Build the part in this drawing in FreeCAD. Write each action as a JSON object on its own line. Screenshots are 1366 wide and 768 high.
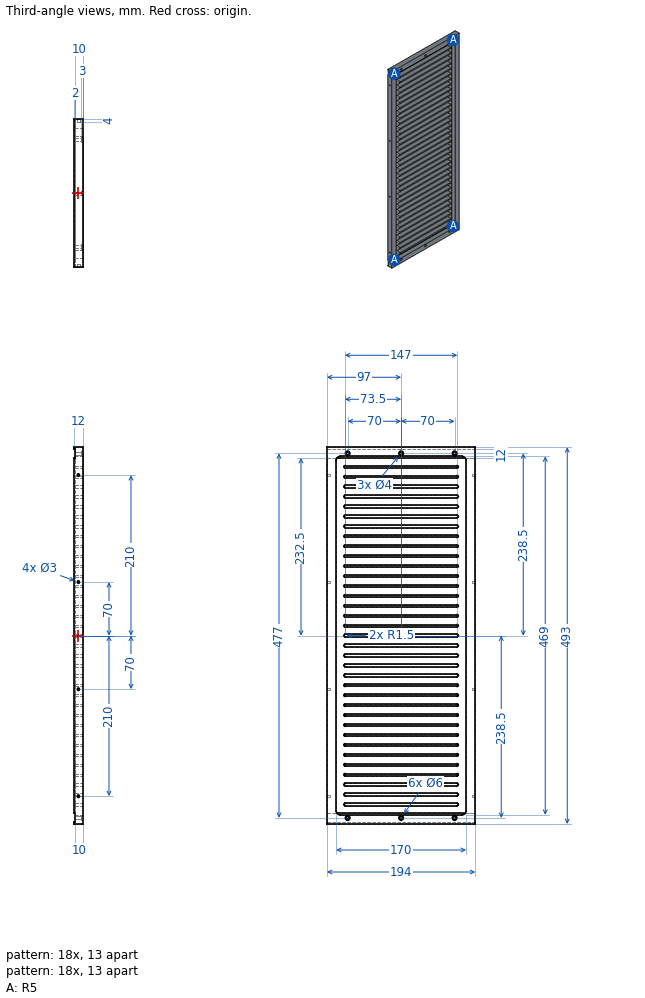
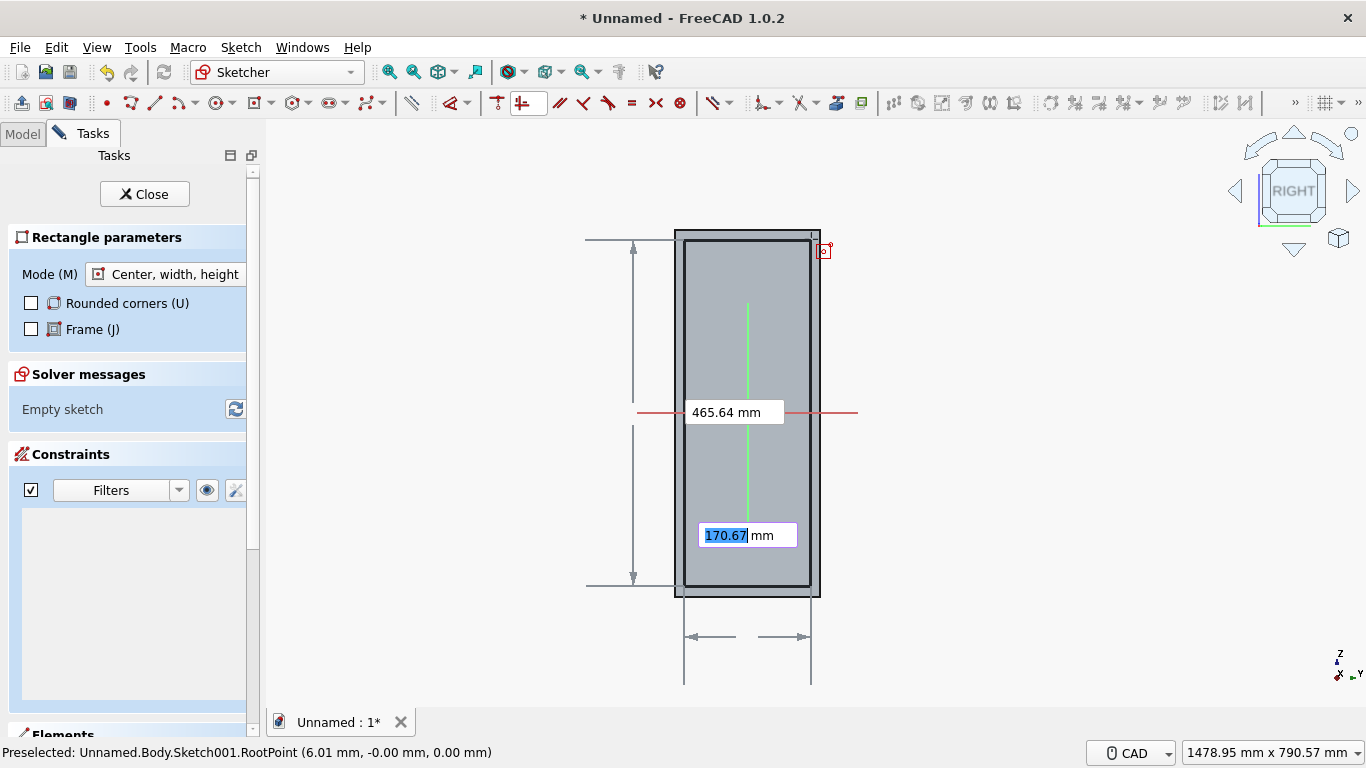
{"action": "type", "text": "170"}
{"action": "key", "text": "Tab"}
{"action": "type", "text": "469"}
{"action": "key", "text": "Return"}
{"action": "key", "text": "Escape"}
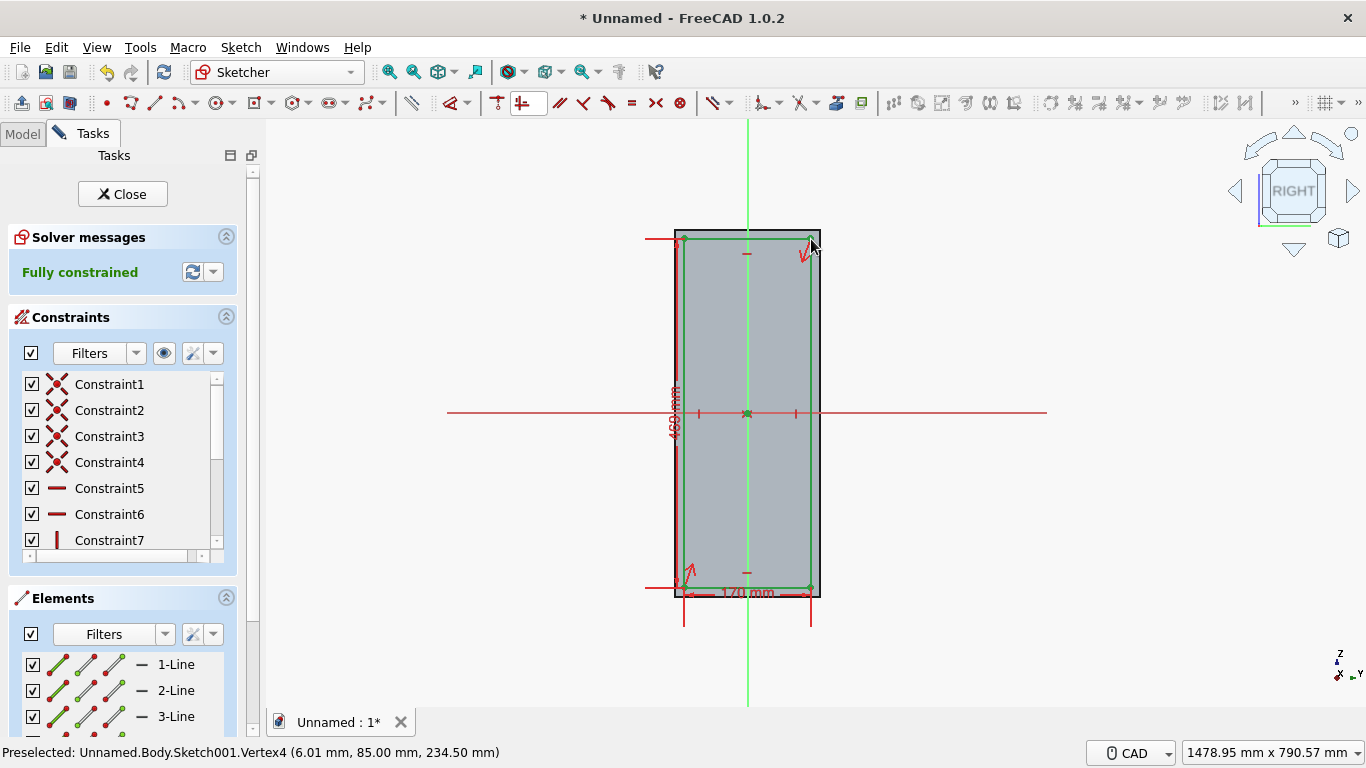
{"action": "left_click", "coordinate": [123, 194]}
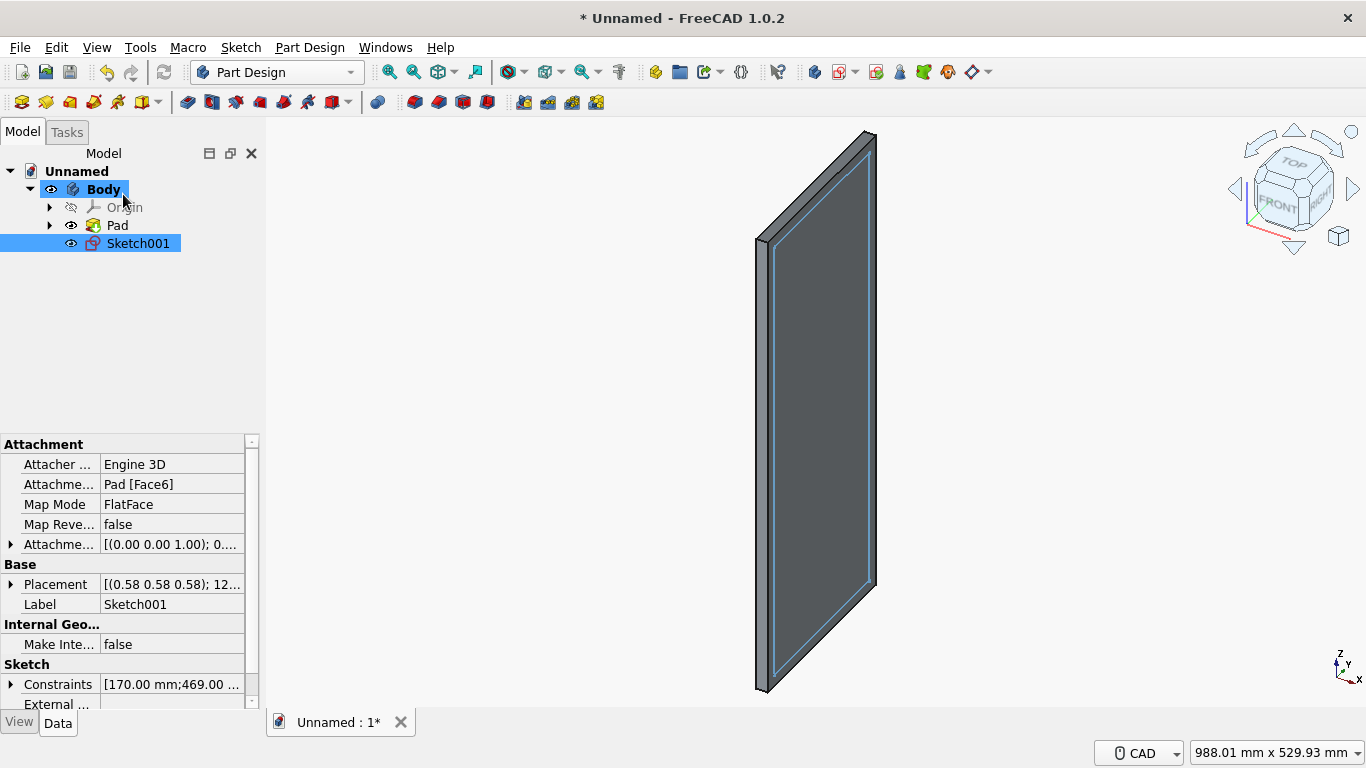
{"action": "left_click", "coordinate": [188, 102]}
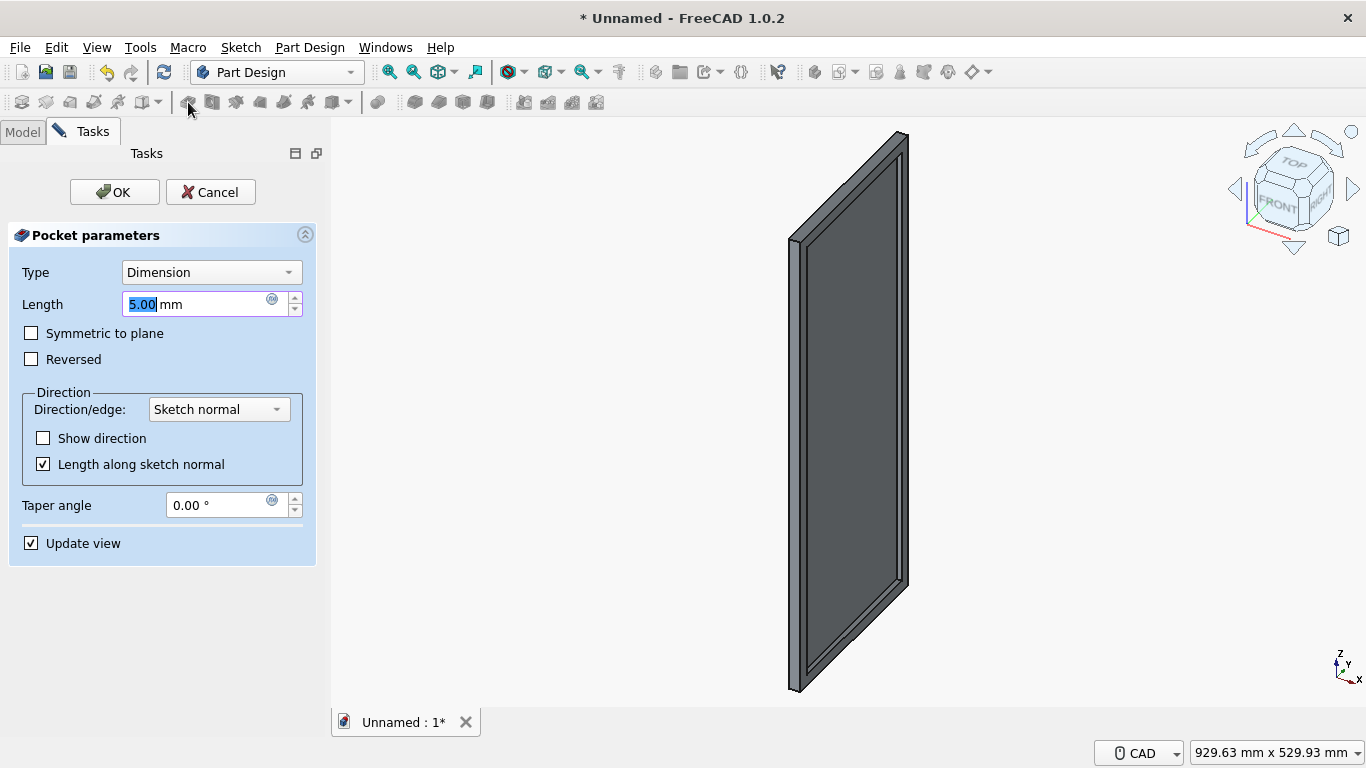
{"action": "type", "text": "10"}
{"action": "key", "text": "Tab"}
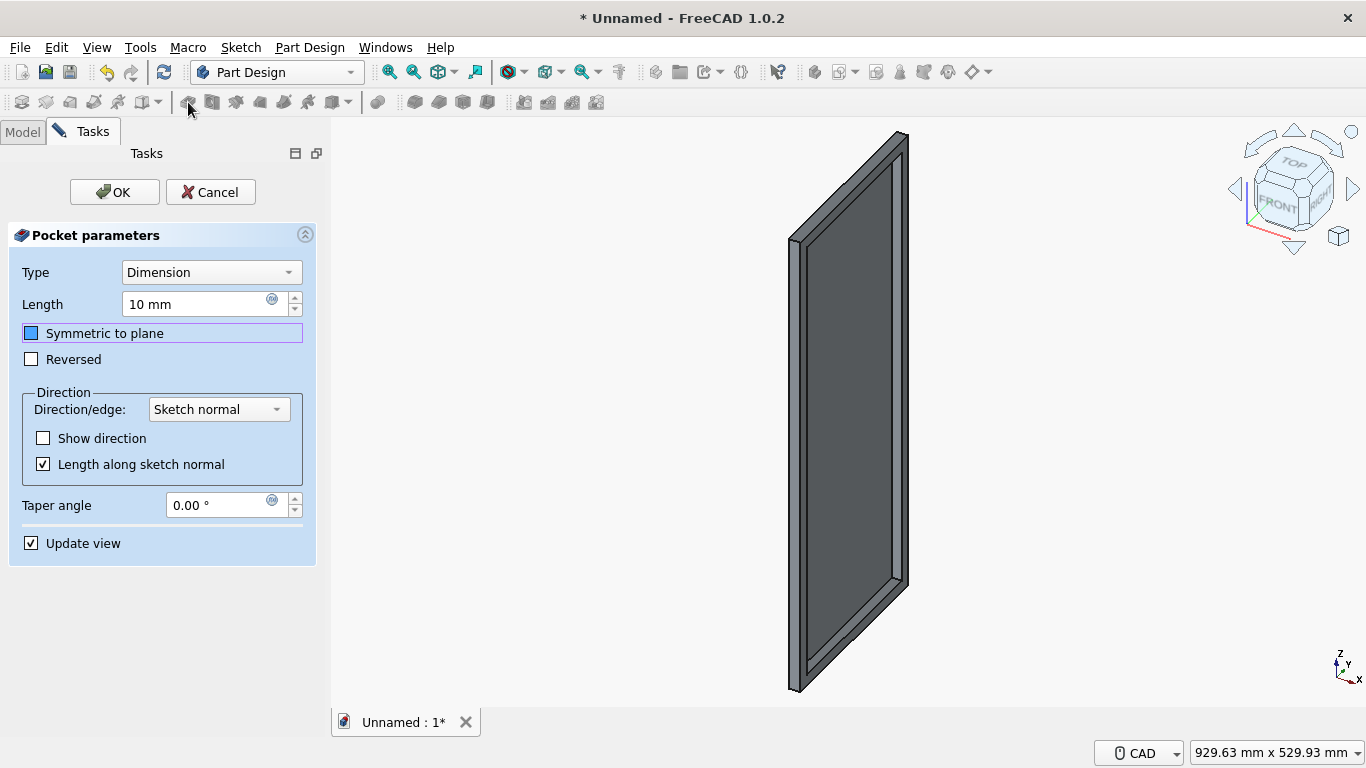
{"action": "left_click", "coordinate": [115, 192]}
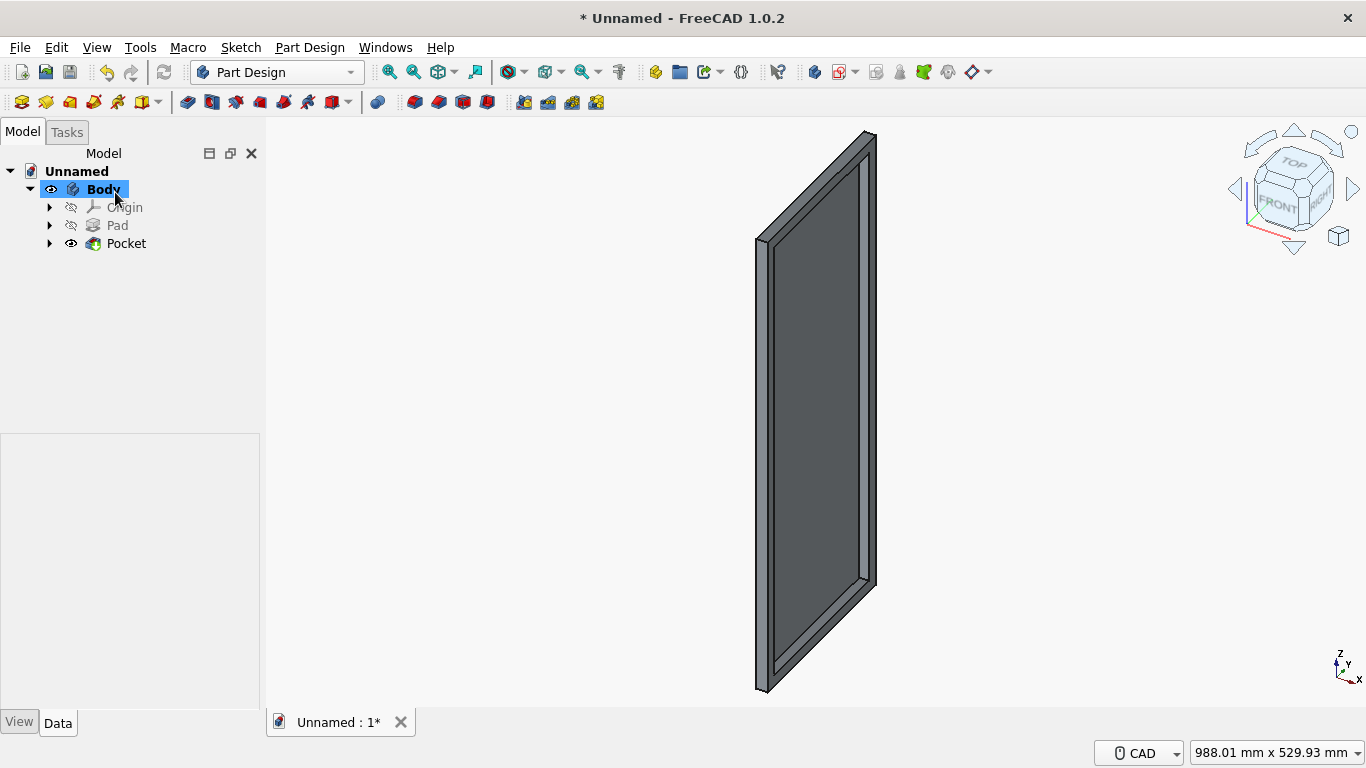
{"action": "left_click", "coordinate": [812, 532]}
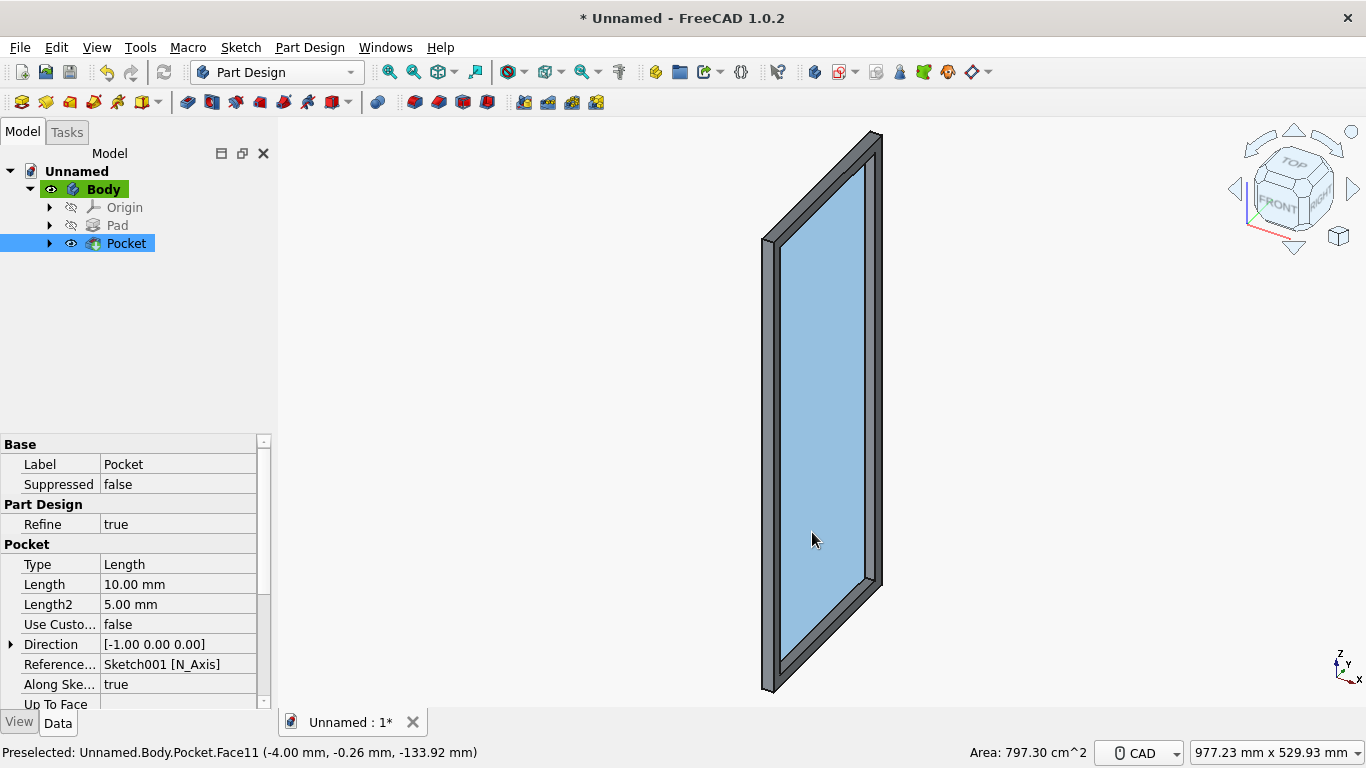
{"action": "left_click", "coordinate": [840, 72]}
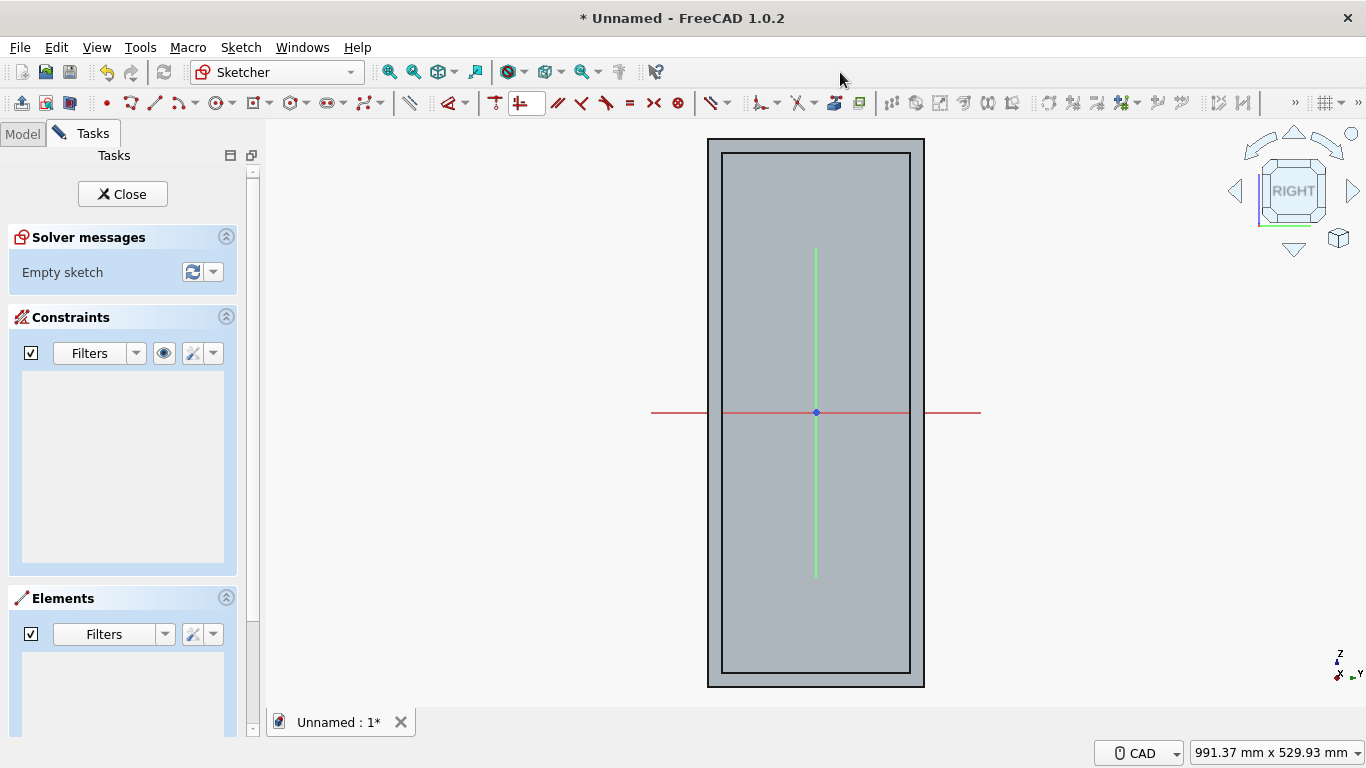
{"action": "scroll", "coordinate": [838, 413], "scroll_direction": "up", "scroll_amount": 7}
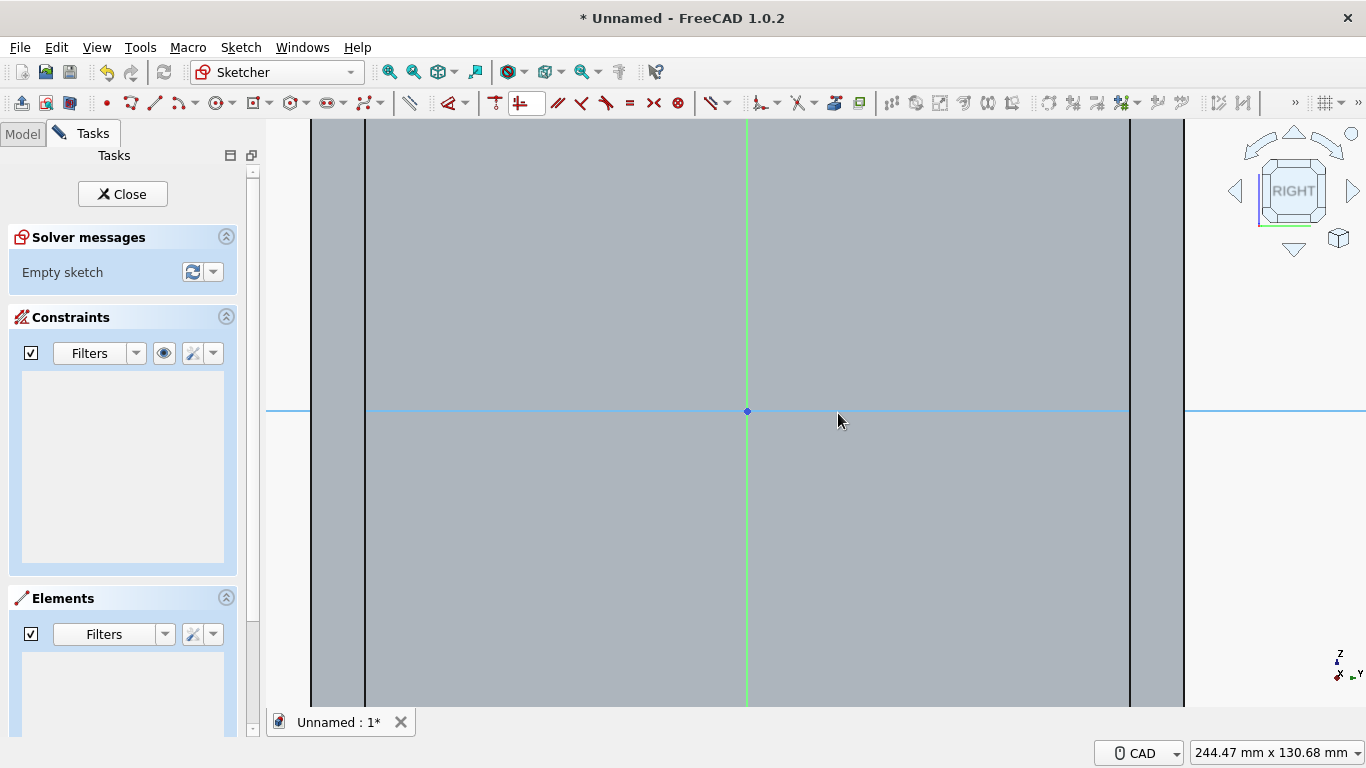
{"action": "left_click", "coordinate": [328, 104]}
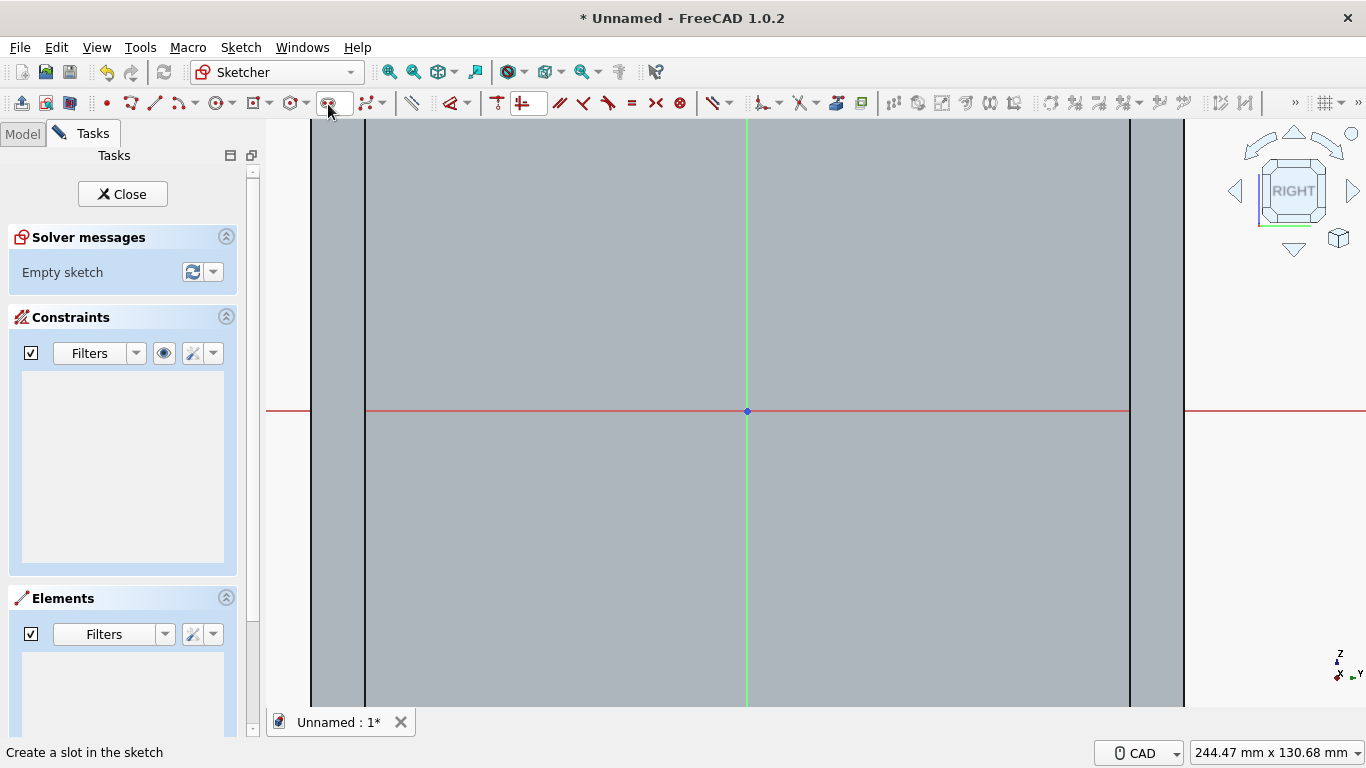
{"action": "scroll", "coordinate": [416, 411], "scroll_direction": "up", "scroll_amount": 7}